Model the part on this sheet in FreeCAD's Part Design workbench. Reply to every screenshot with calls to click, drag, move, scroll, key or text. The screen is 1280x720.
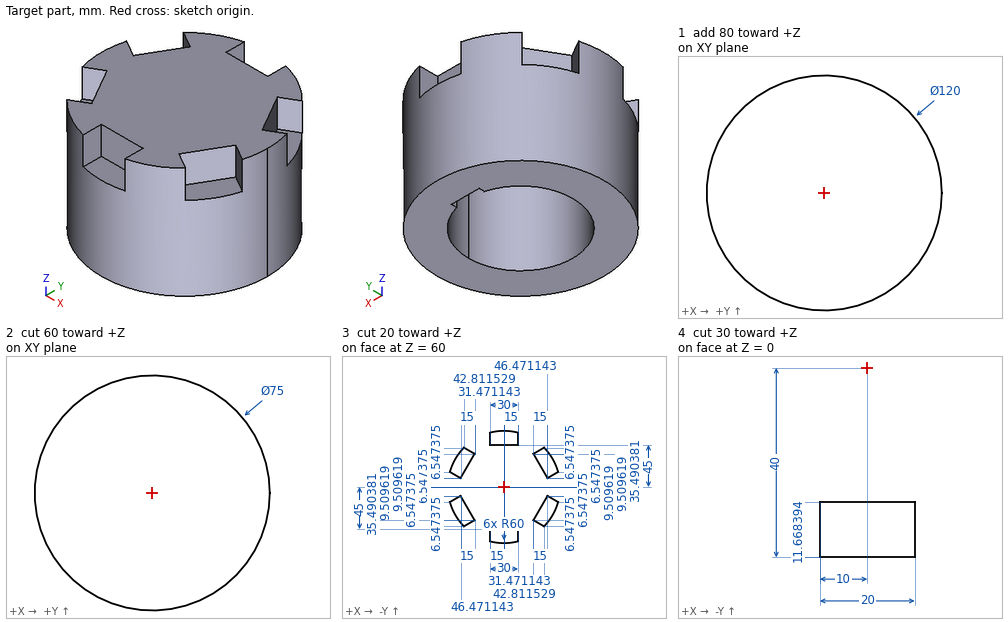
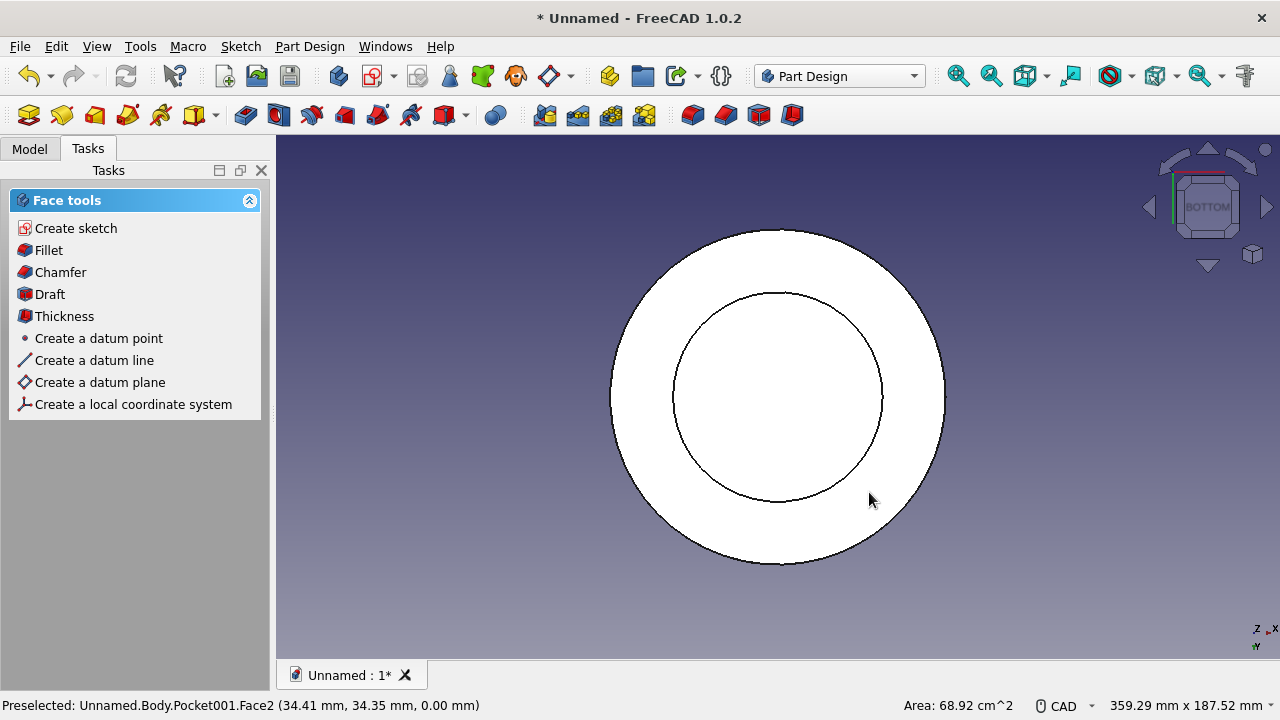
click(372, 76)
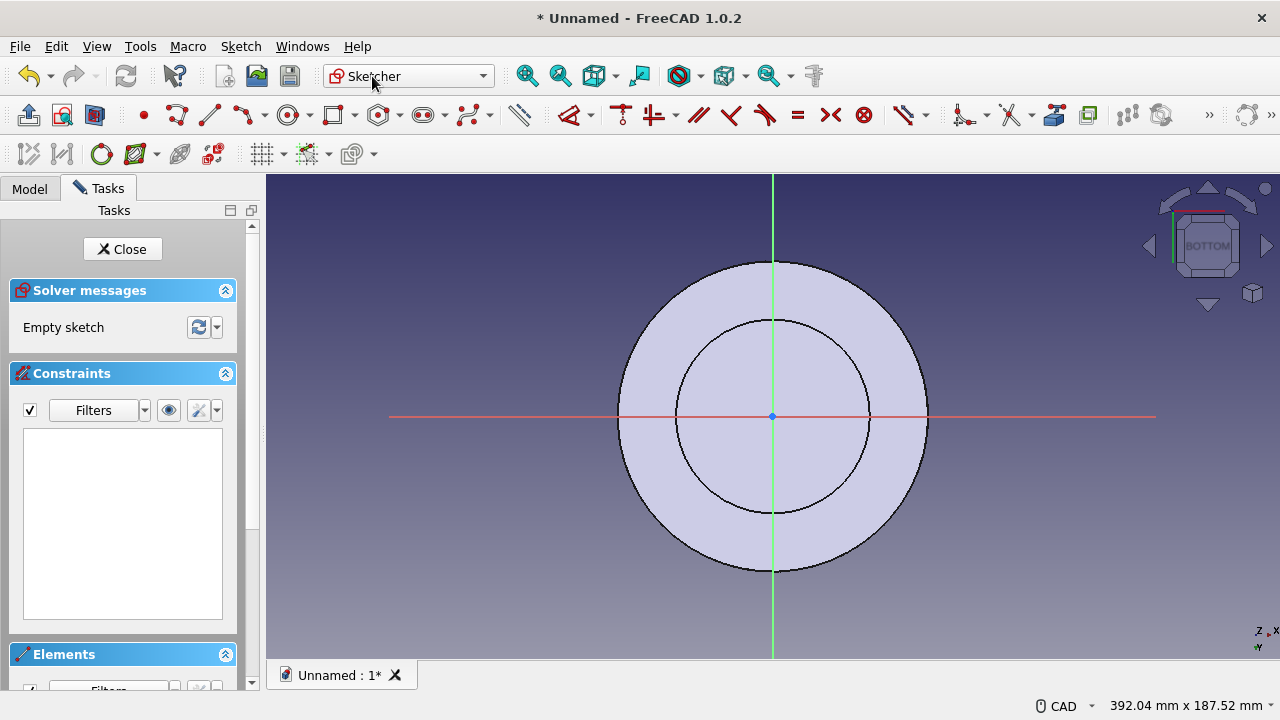
scroll(813, 498, up, 5)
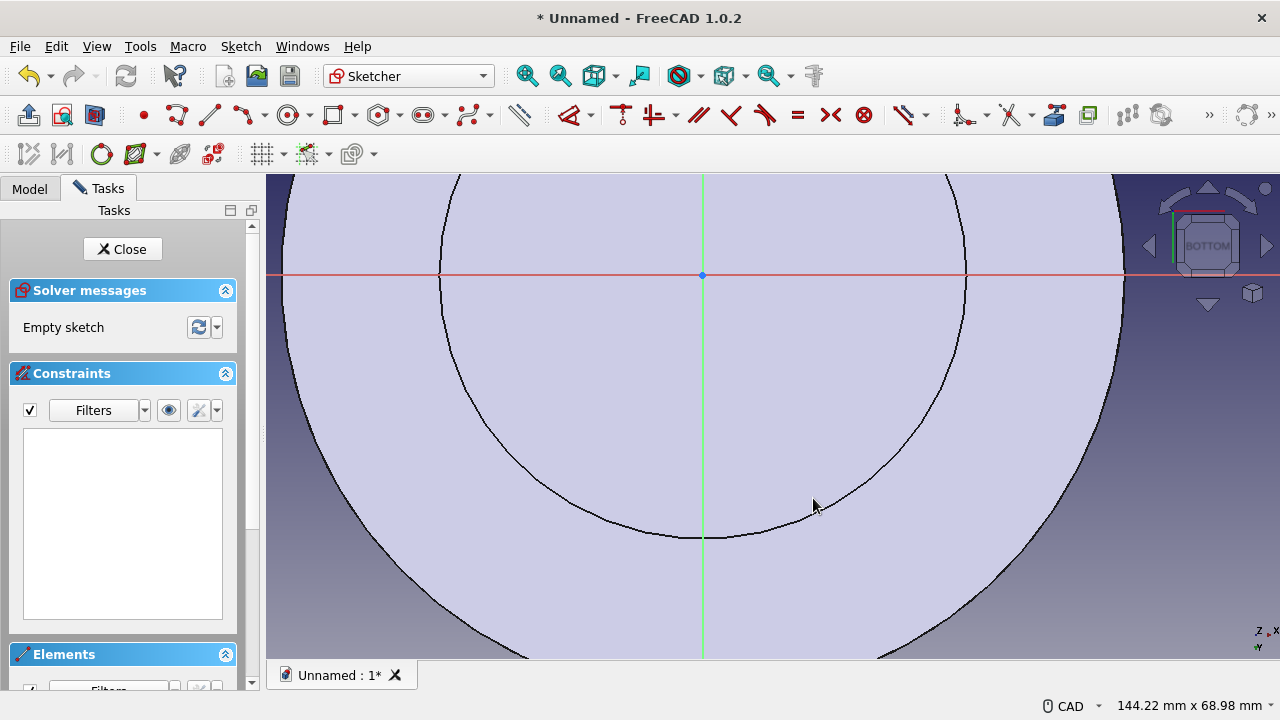
click(332, 116)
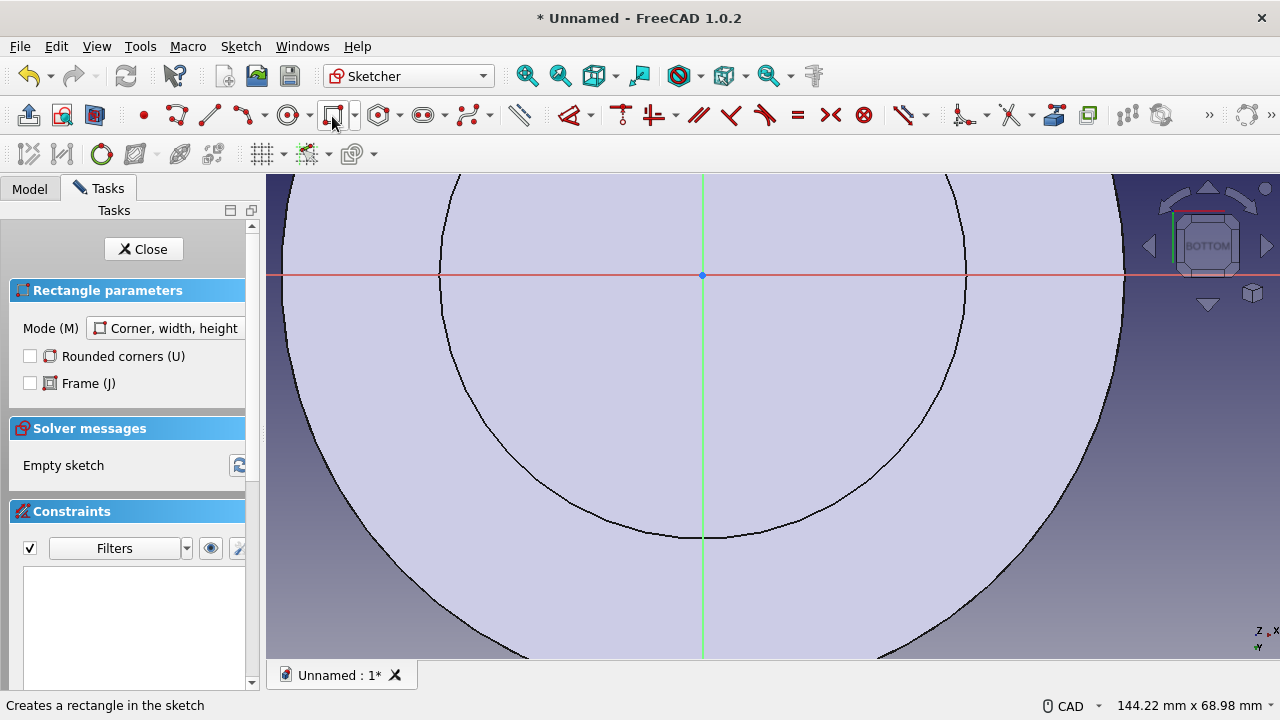
click(633, 475)
click(773, 557)
key(Escape)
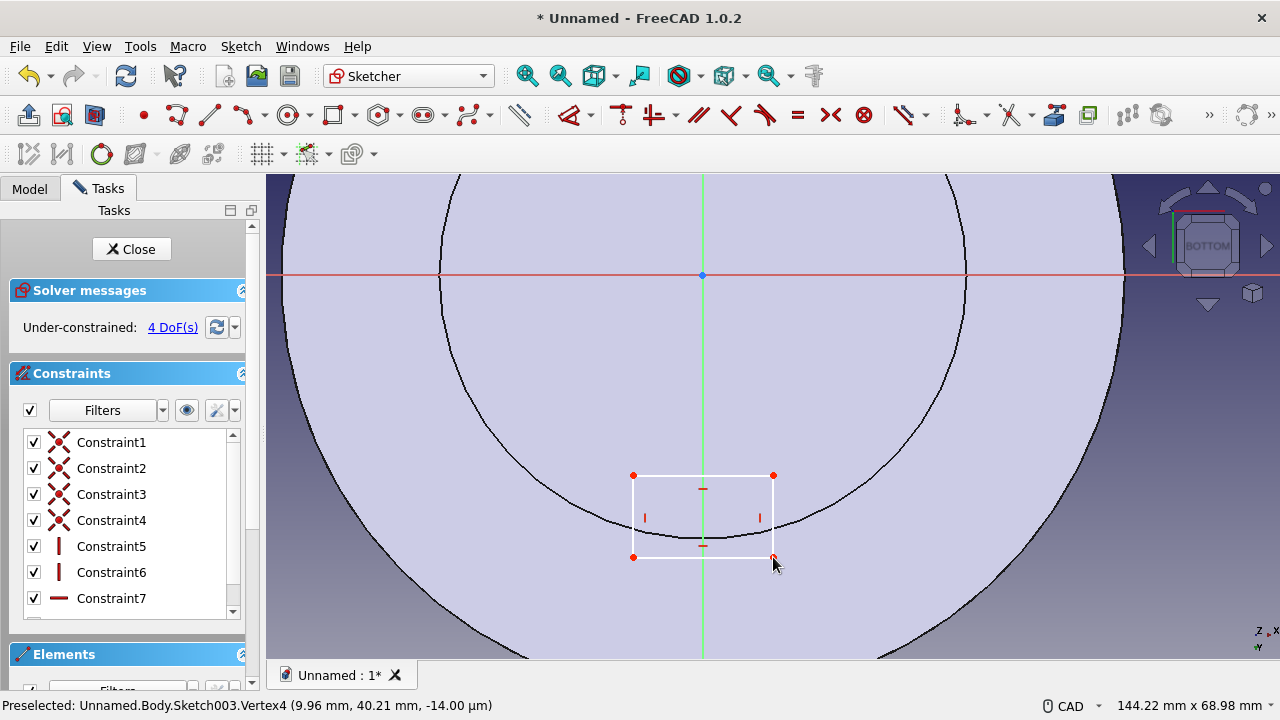
click(568, 116)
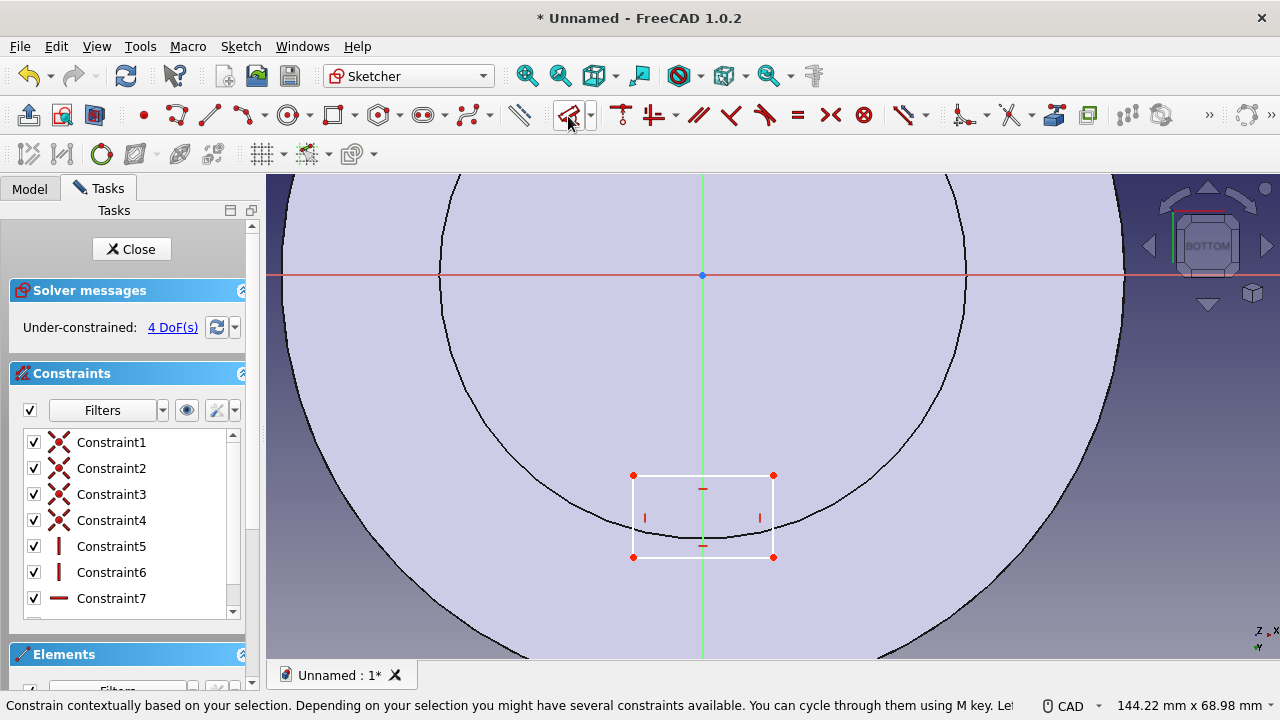
click(675, 558)
click(671, 592)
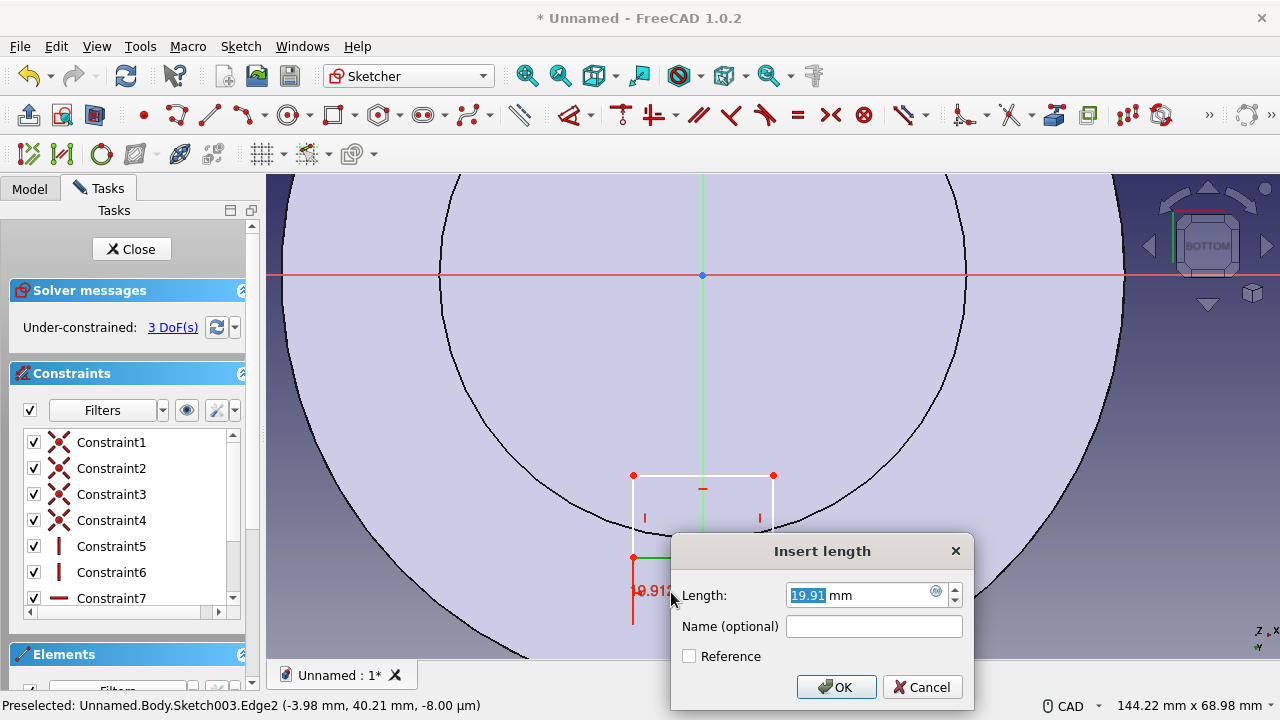
text(20)
key(Return)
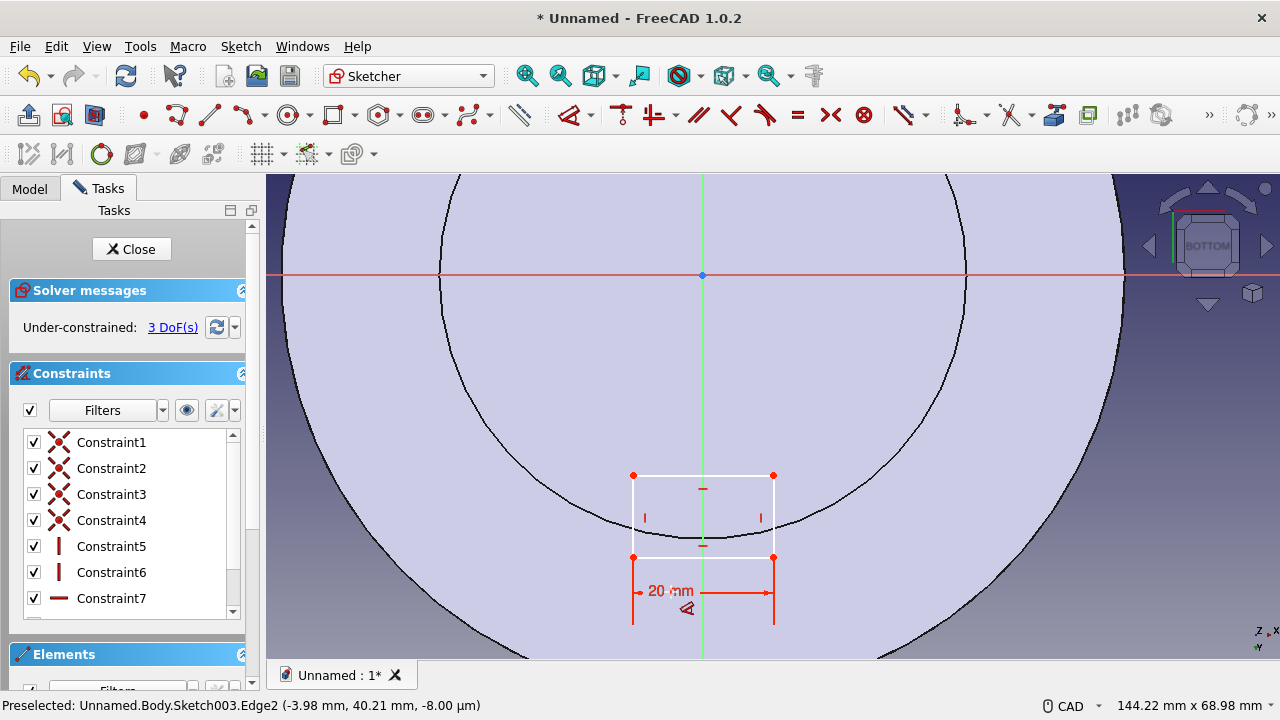
click(633, 476)
click(668, 241)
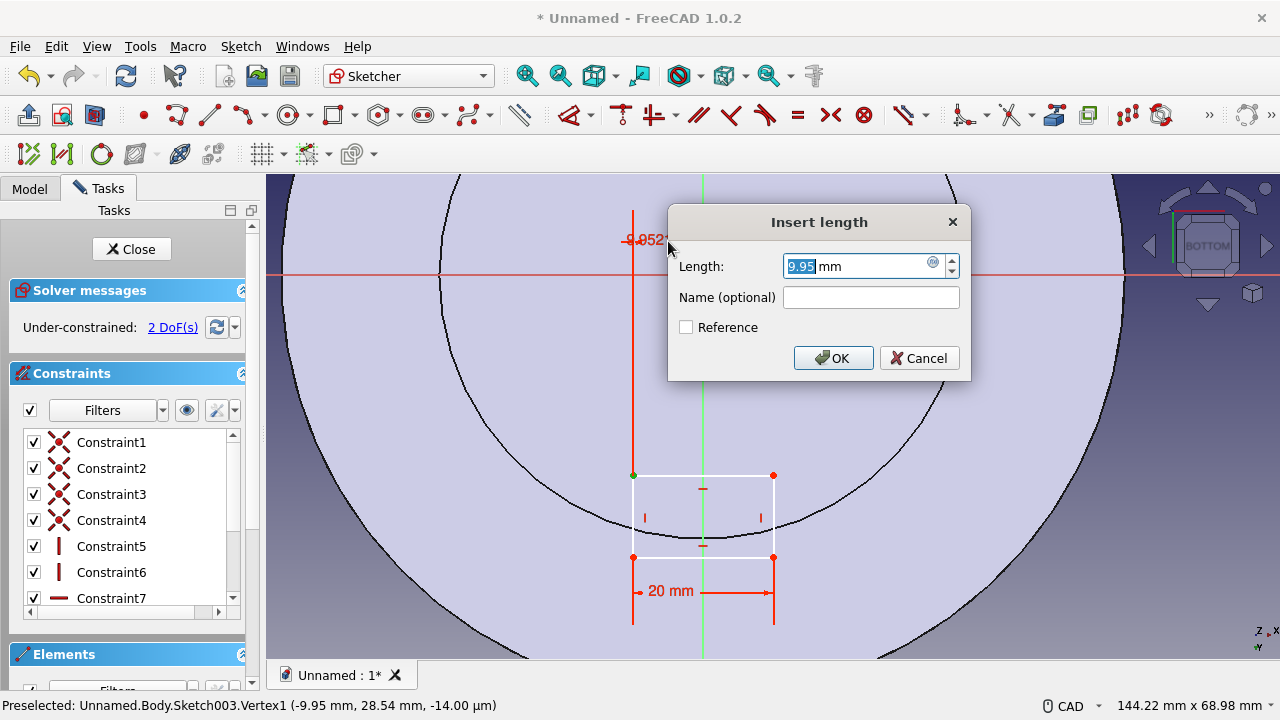
text(10)
key(Return)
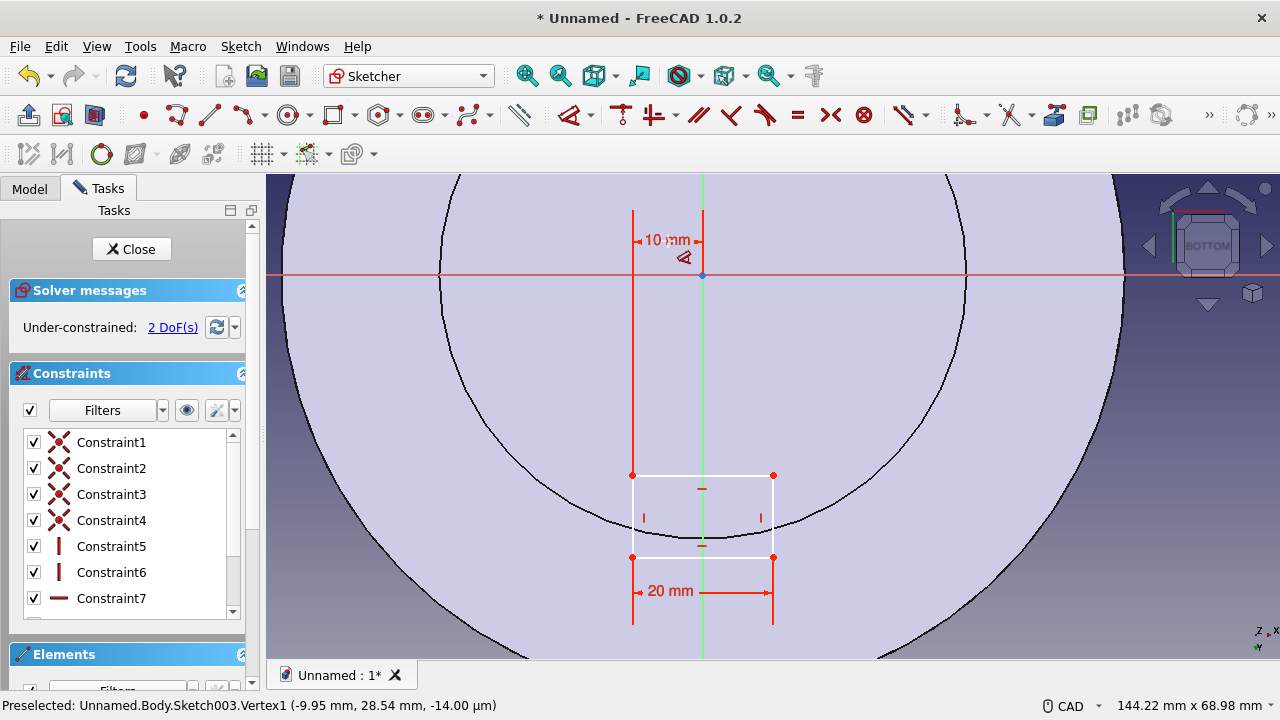
click(633, 558)
click(599, 417)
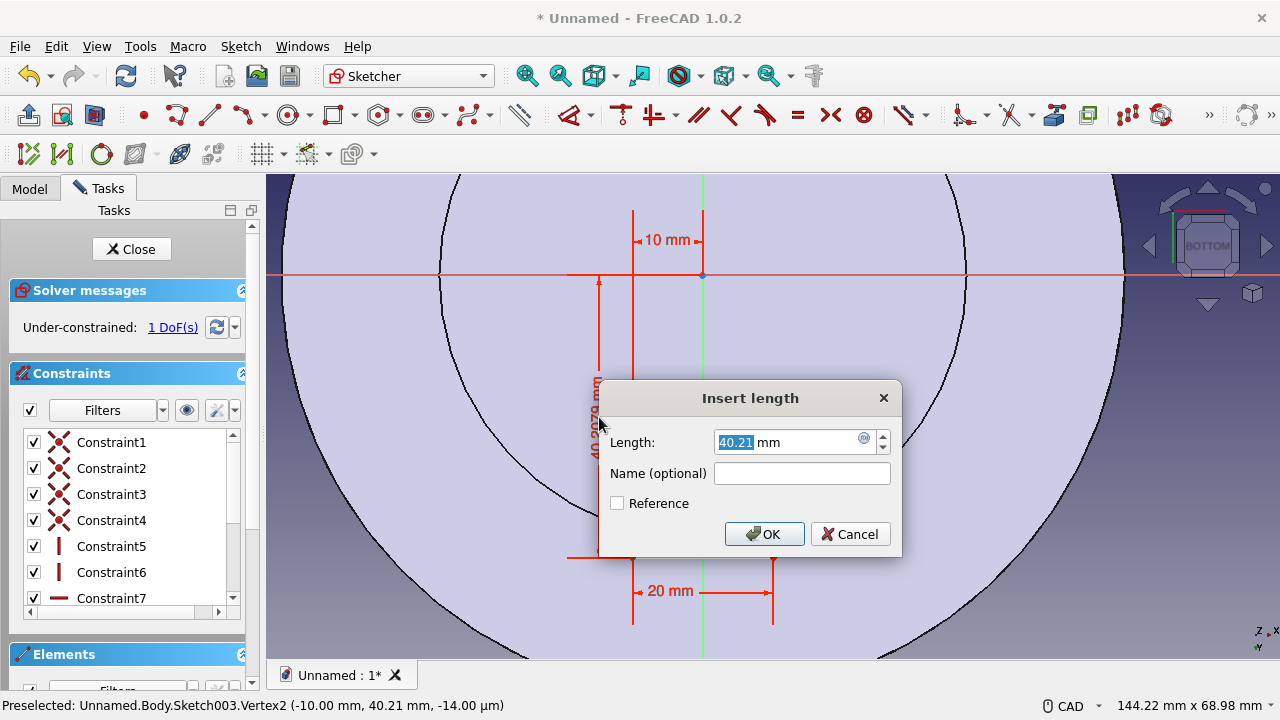
text(40)
key(Return)